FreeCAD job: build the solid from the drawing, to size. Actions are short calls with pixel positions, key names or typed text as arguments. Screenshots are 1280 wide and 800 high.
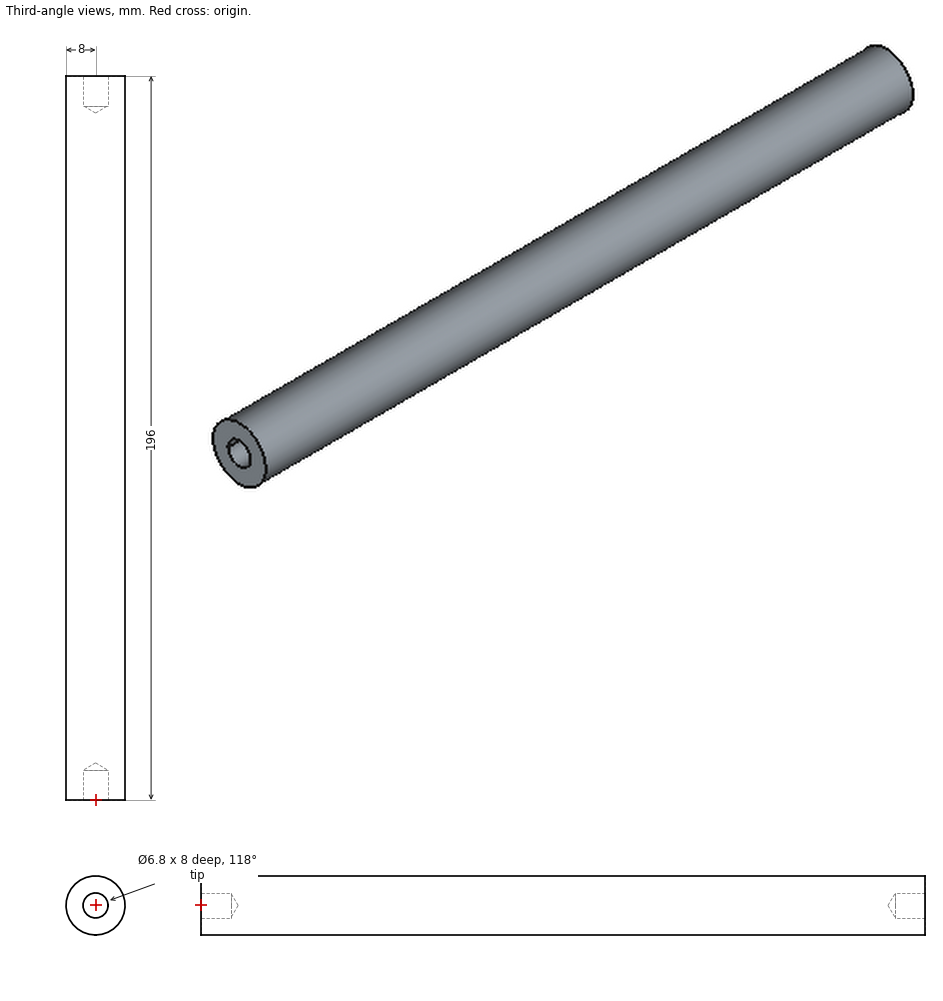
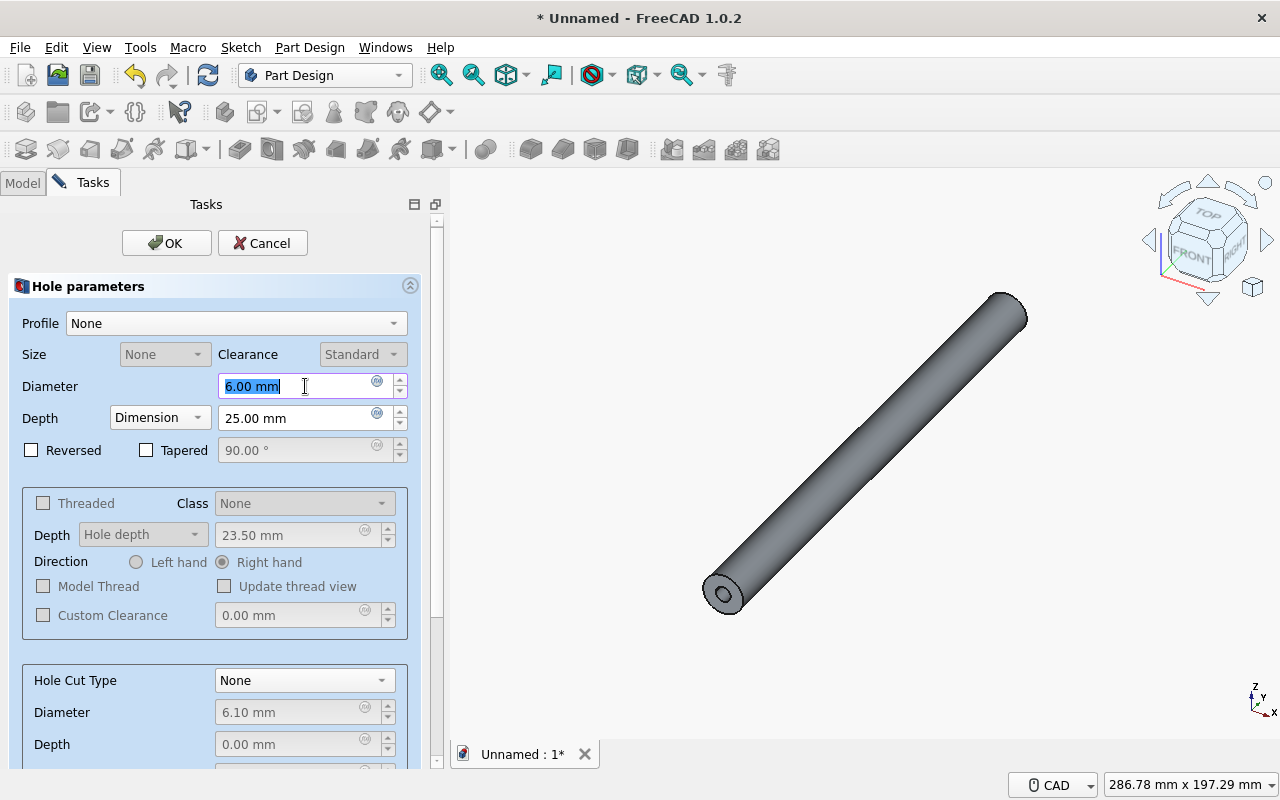
text(6.8)
key(Tab)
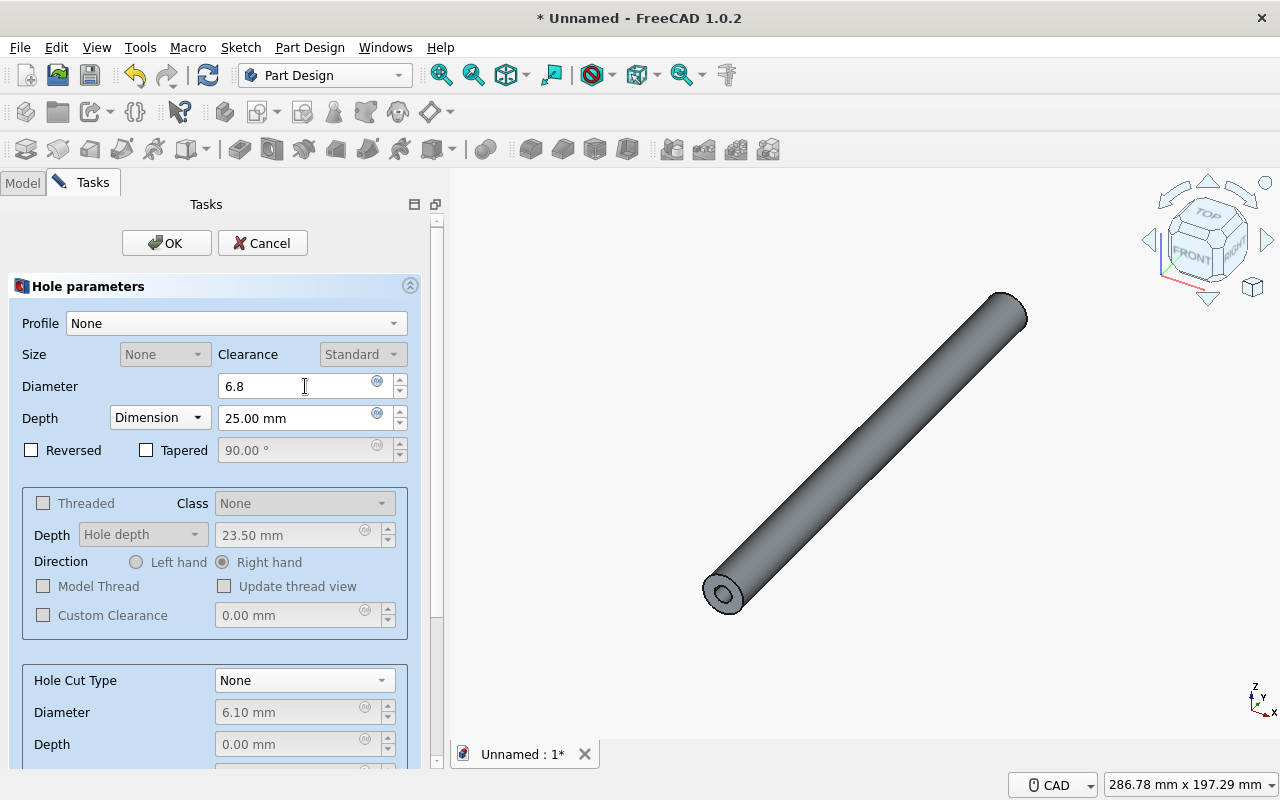
triple_click(305, 418)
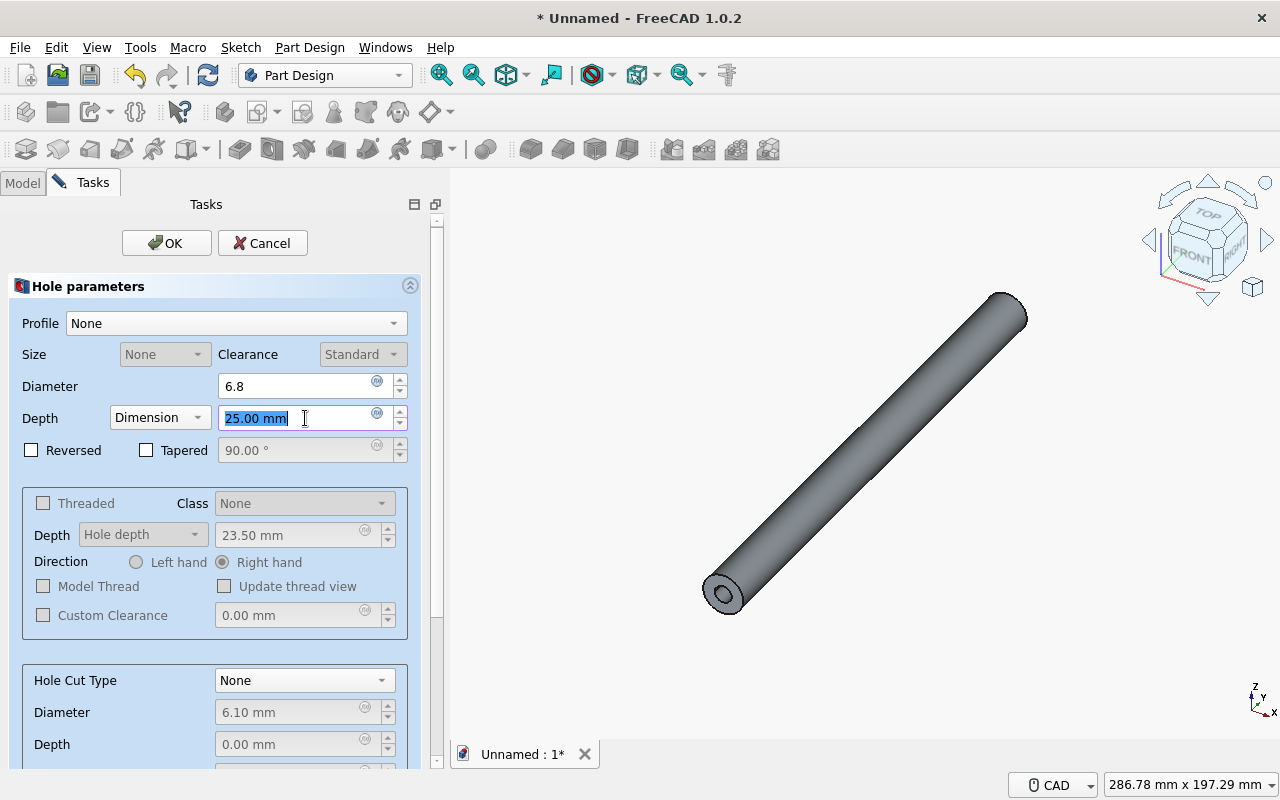
text(8)
key(Tab)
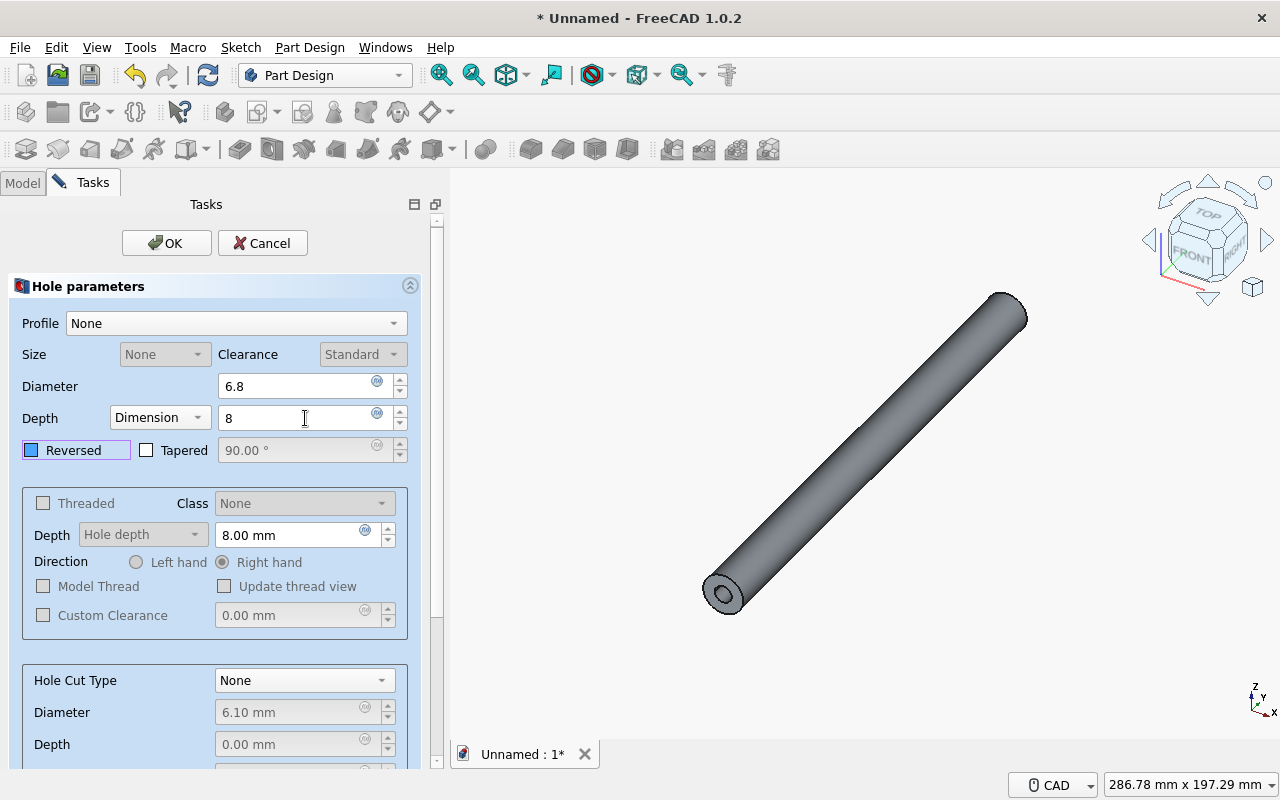
click(167, 243)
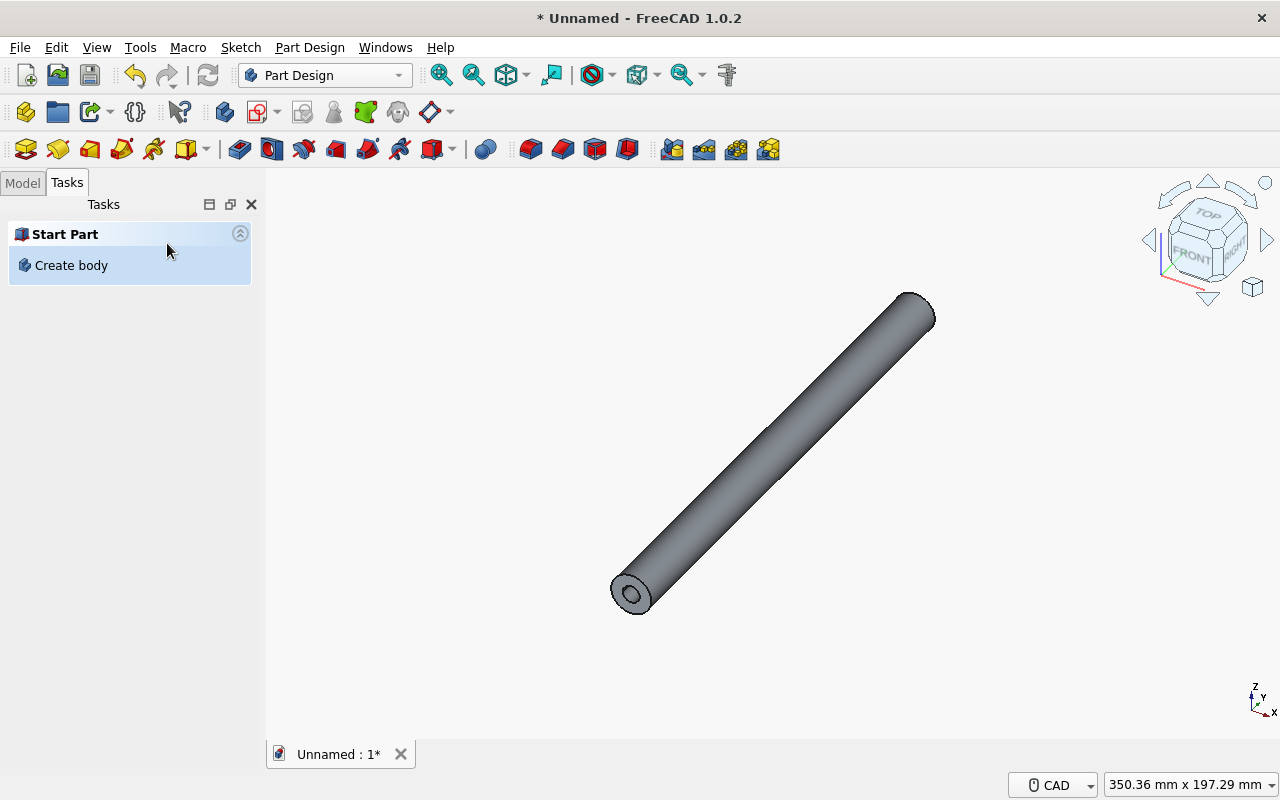
key(4)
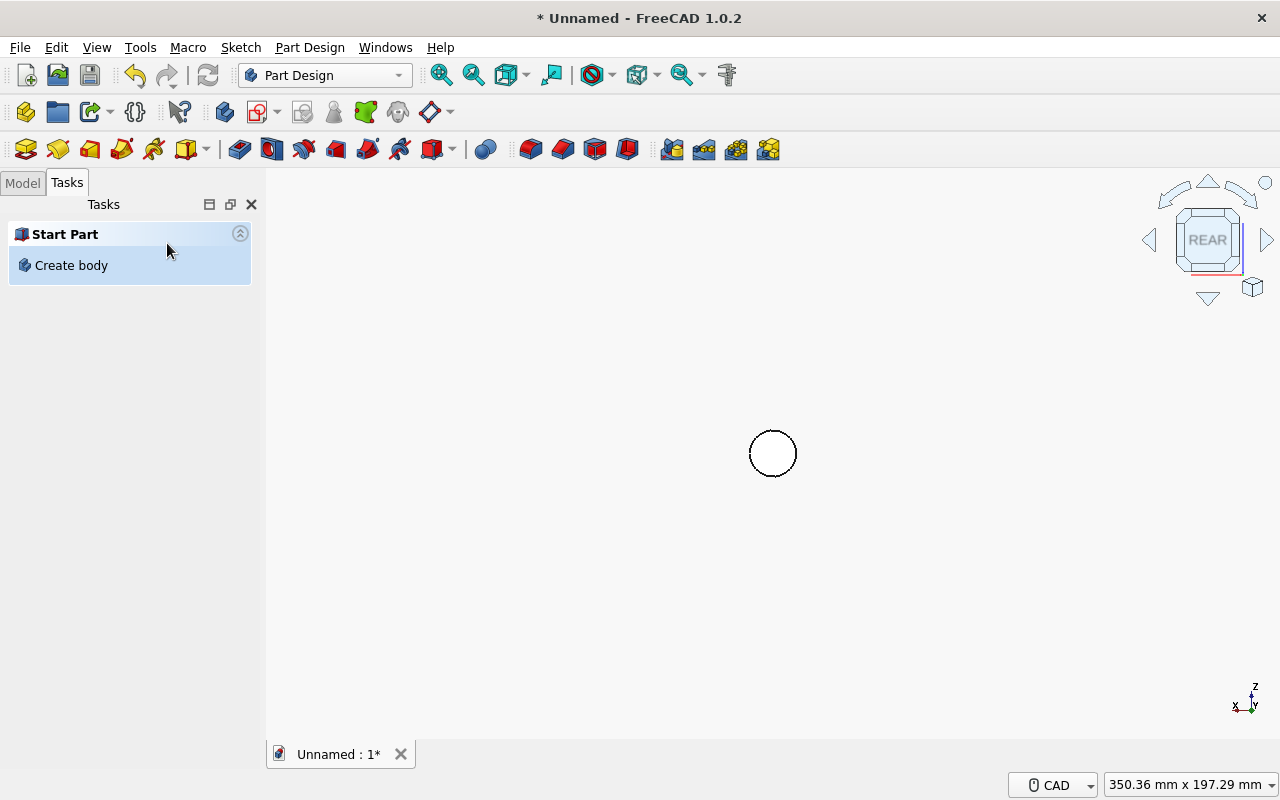
click(442, 76)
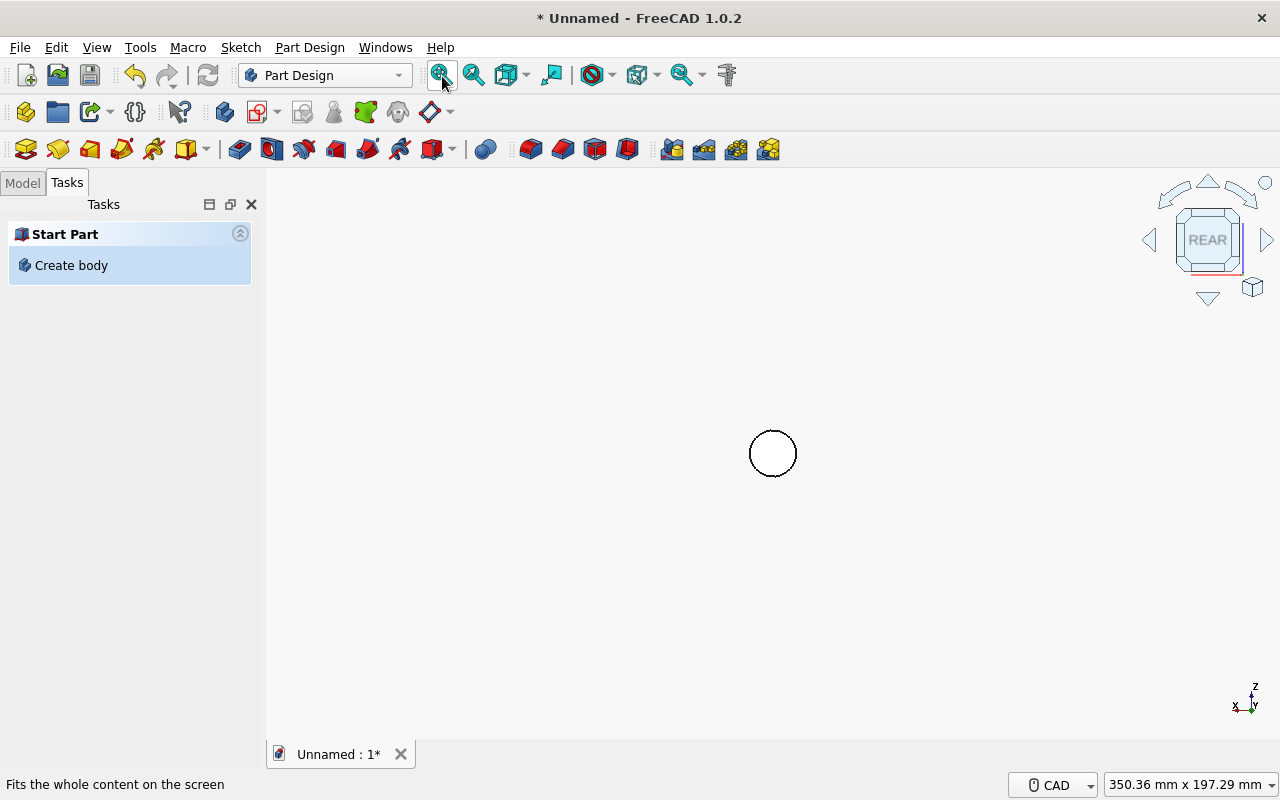
click(773, 453)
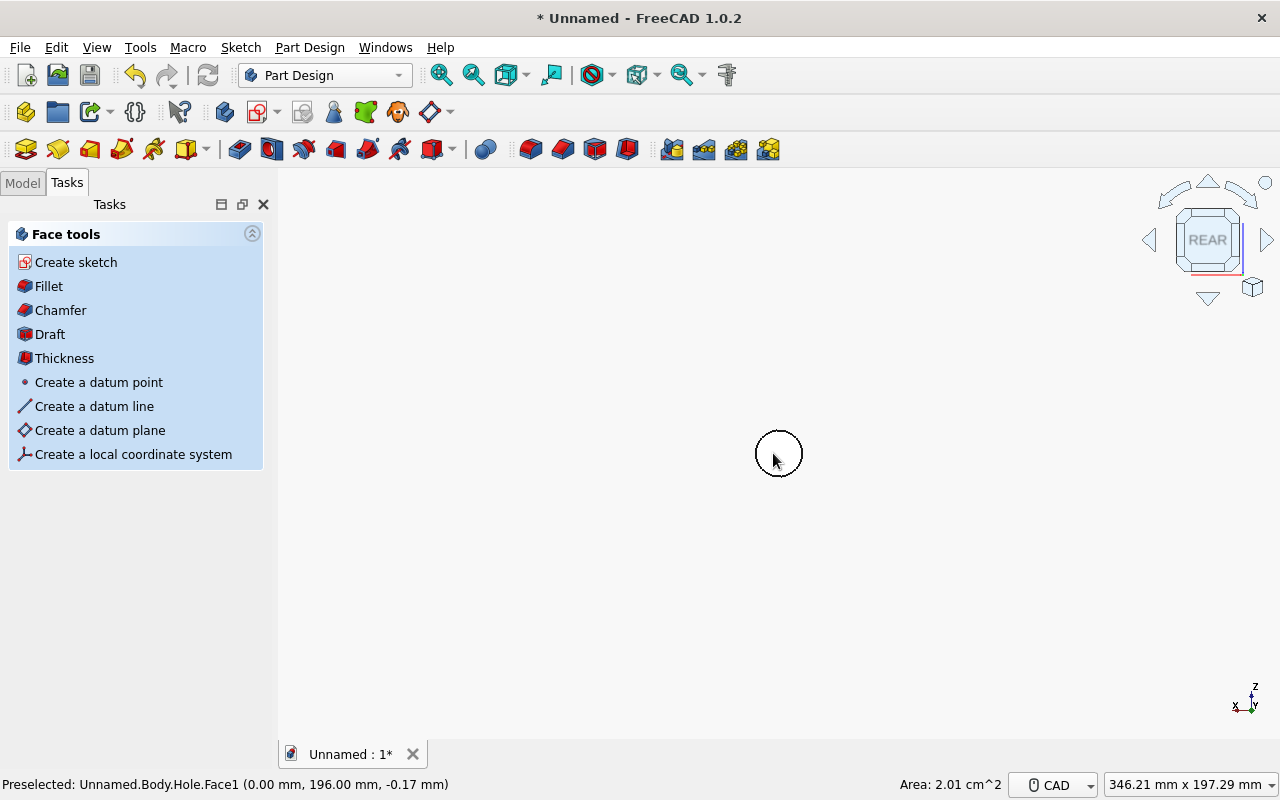
click(258, 112)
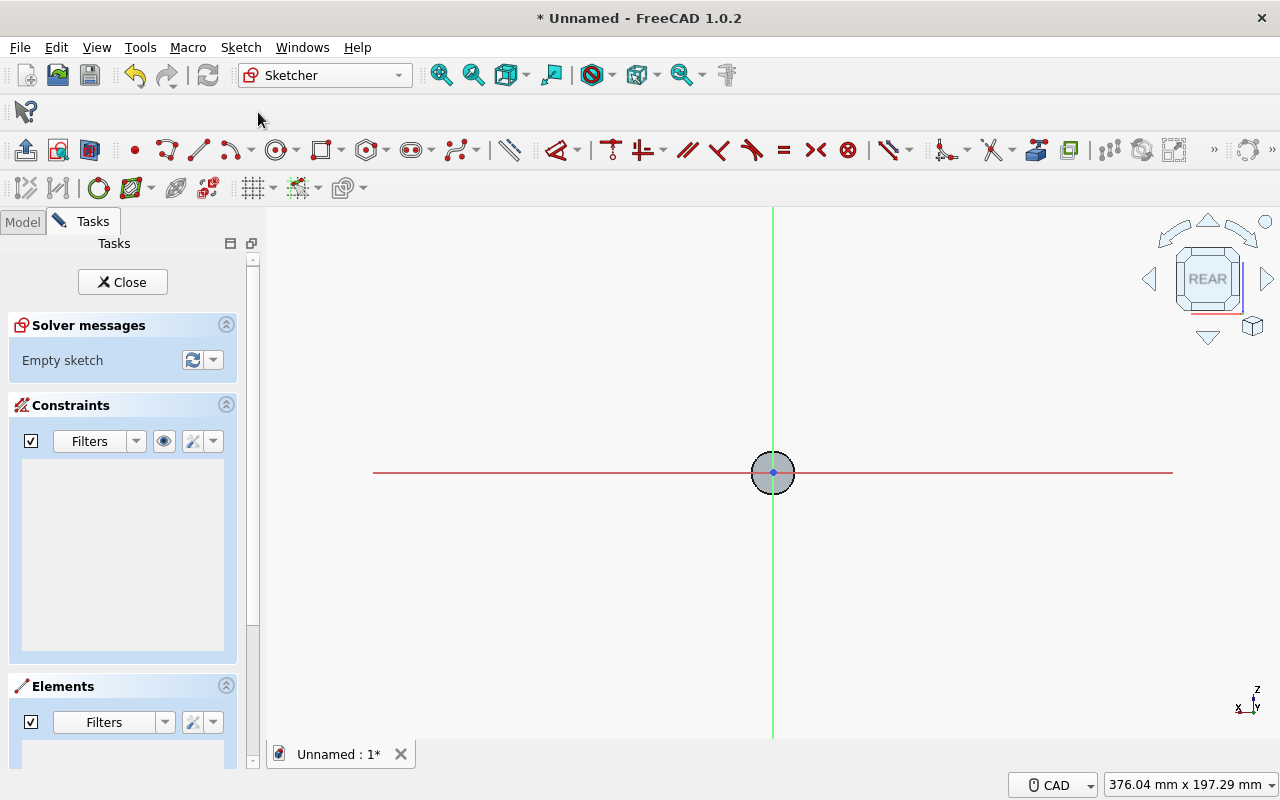
scroll(777, 473, up, 15)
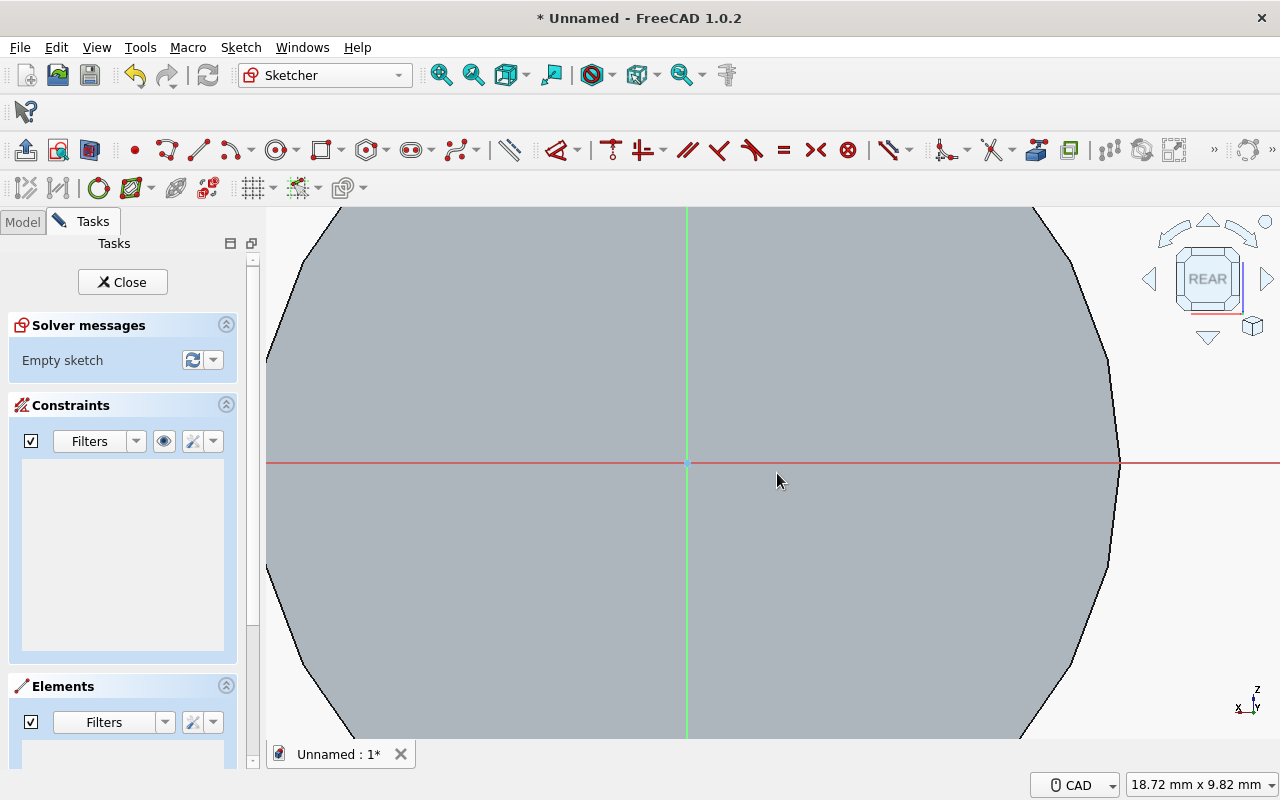
click(276, 150)